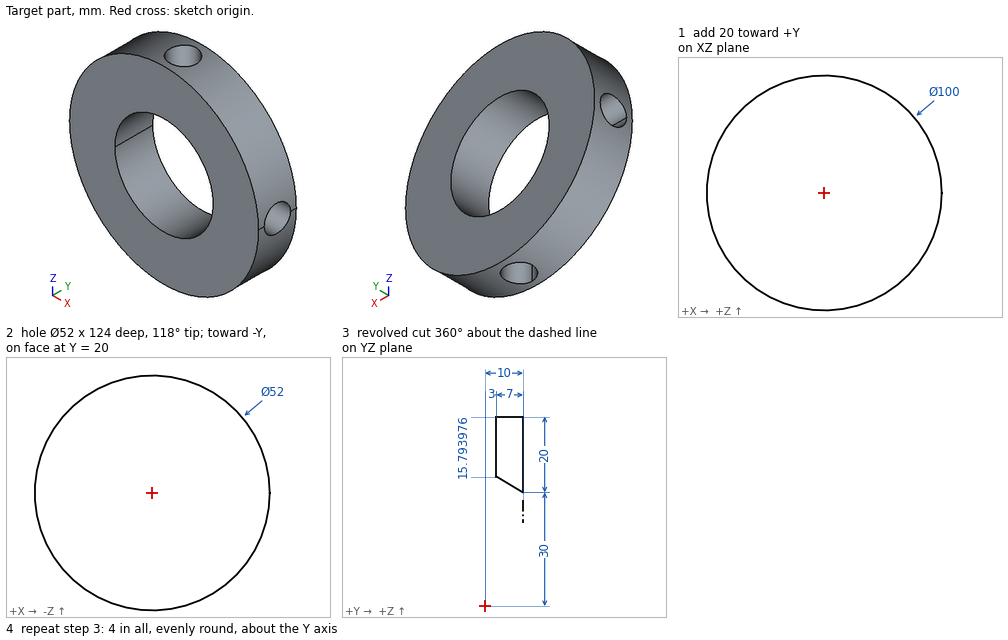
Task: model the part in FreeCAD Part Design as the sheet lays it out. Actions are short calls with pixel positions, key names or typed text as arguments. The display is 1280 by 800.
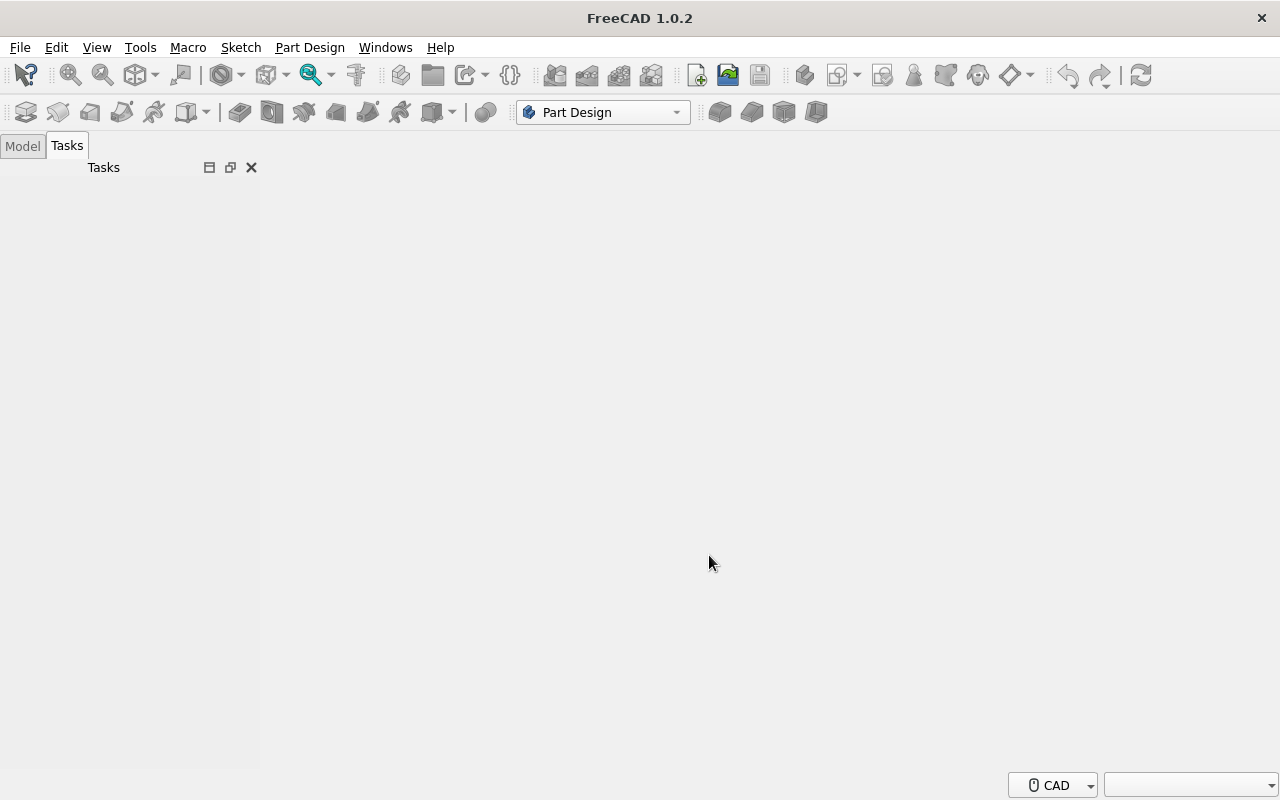
key(ctrl+n)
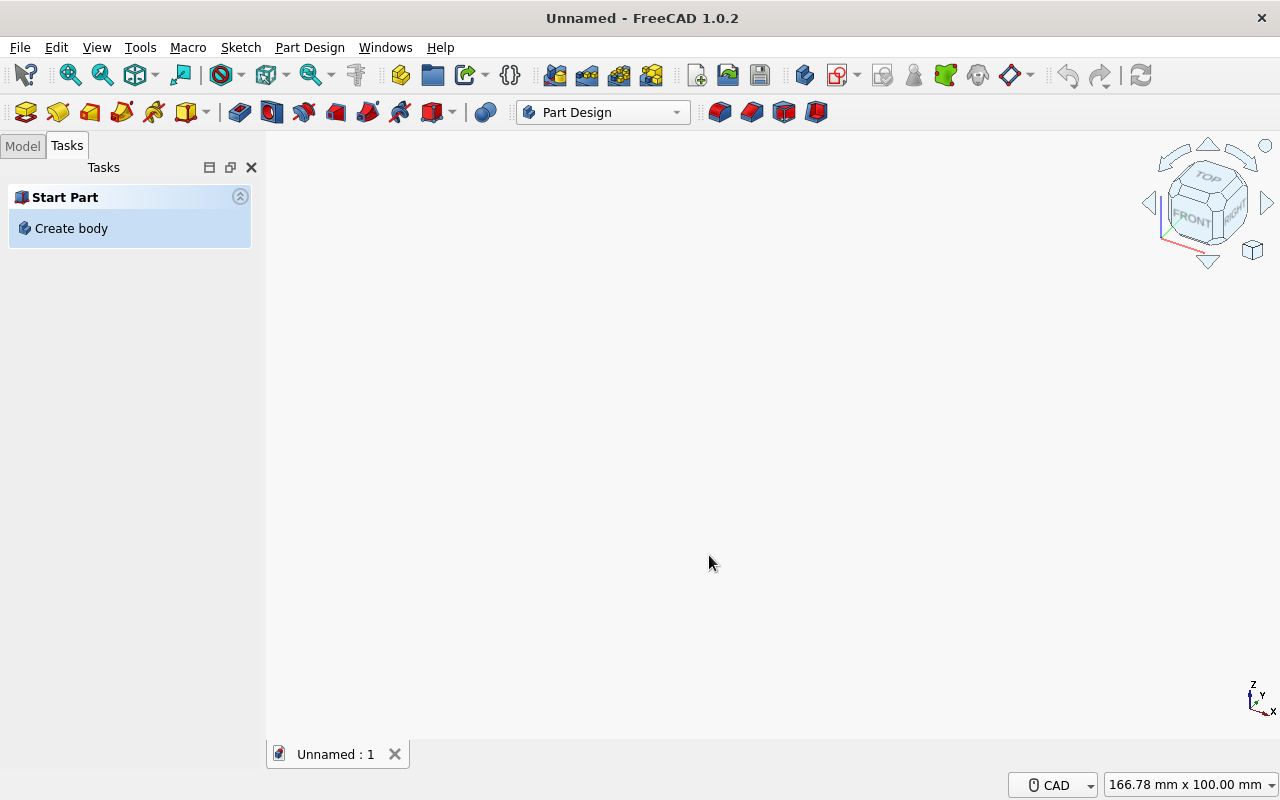
click(838, 76)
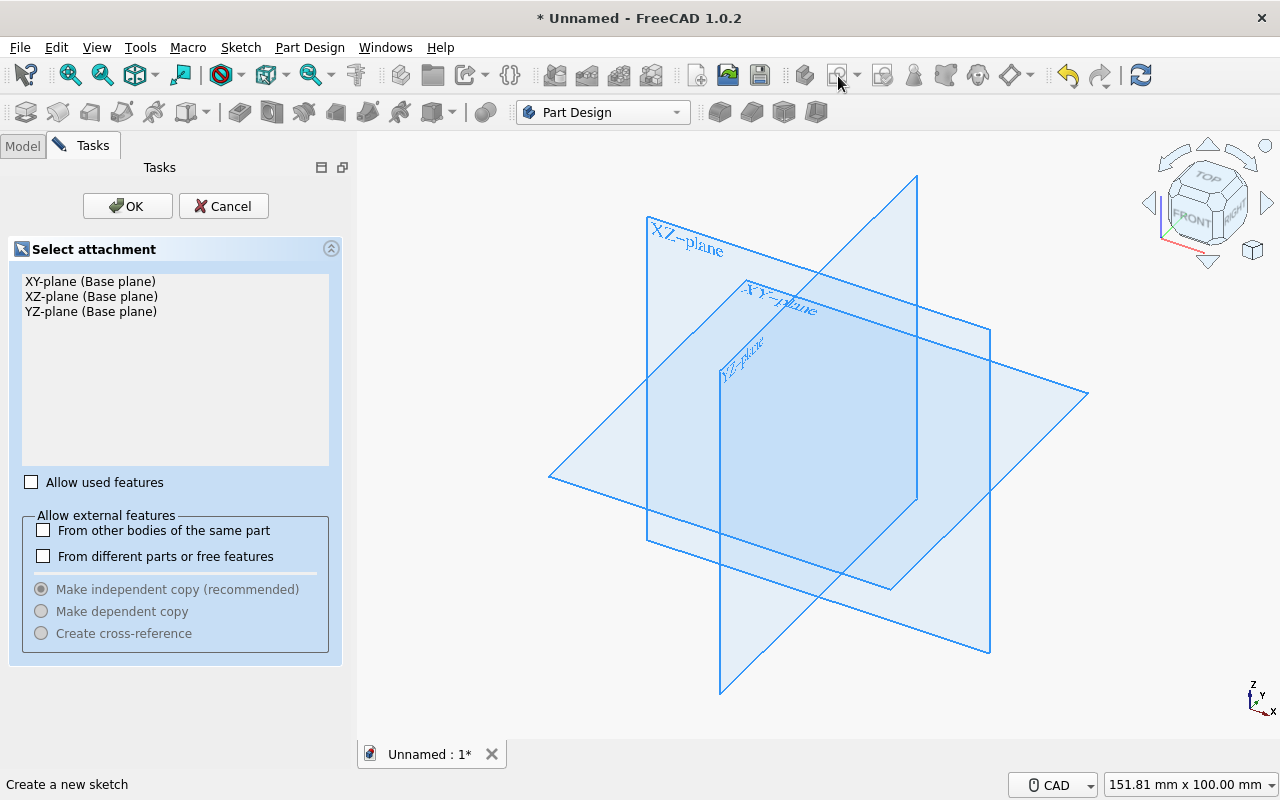
click(82, 296)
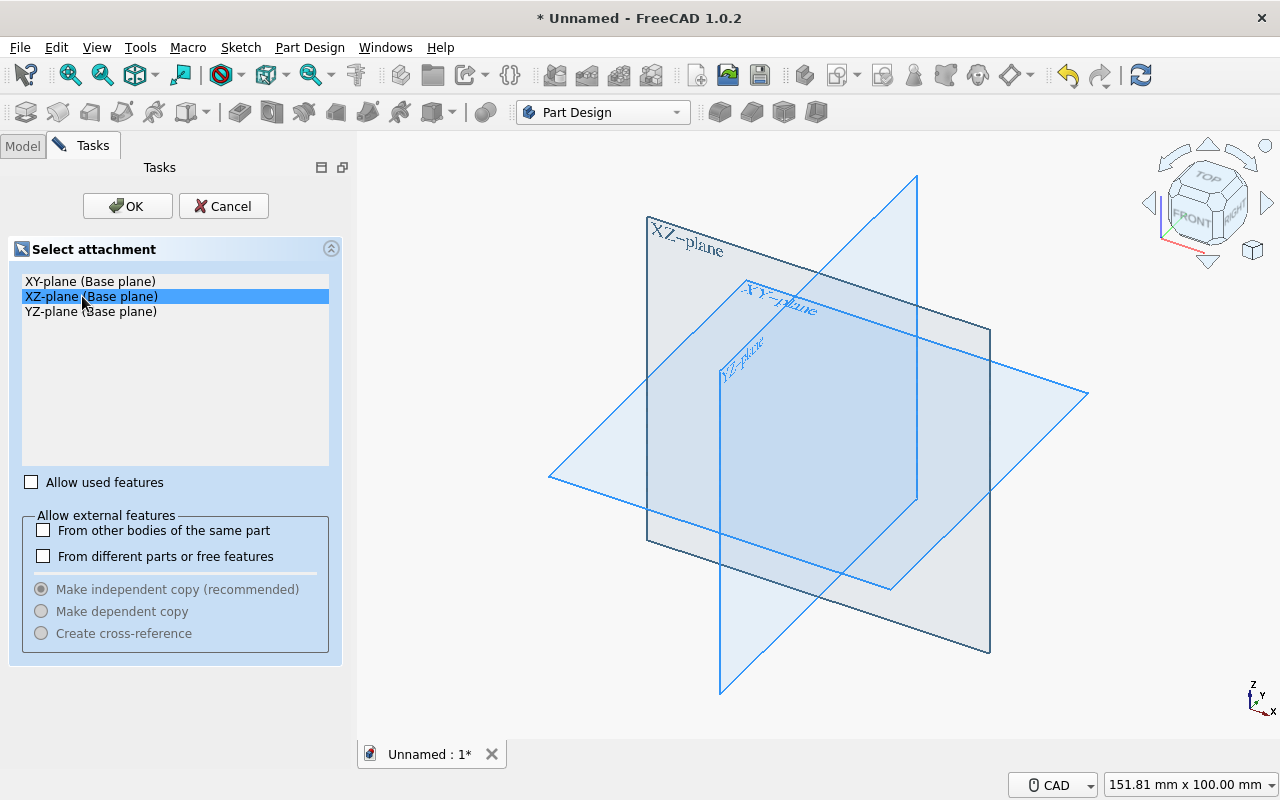
click(128, 206)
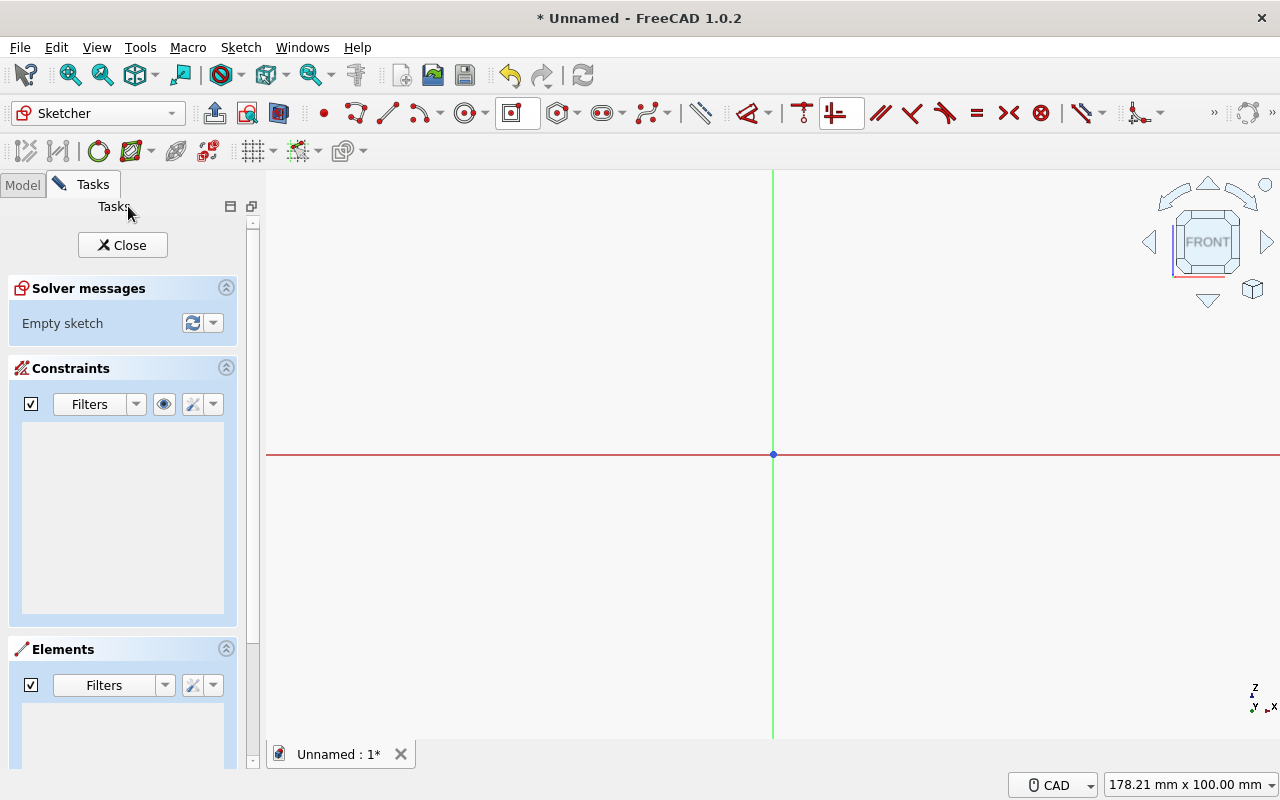
scroll(565, 455, down, 2)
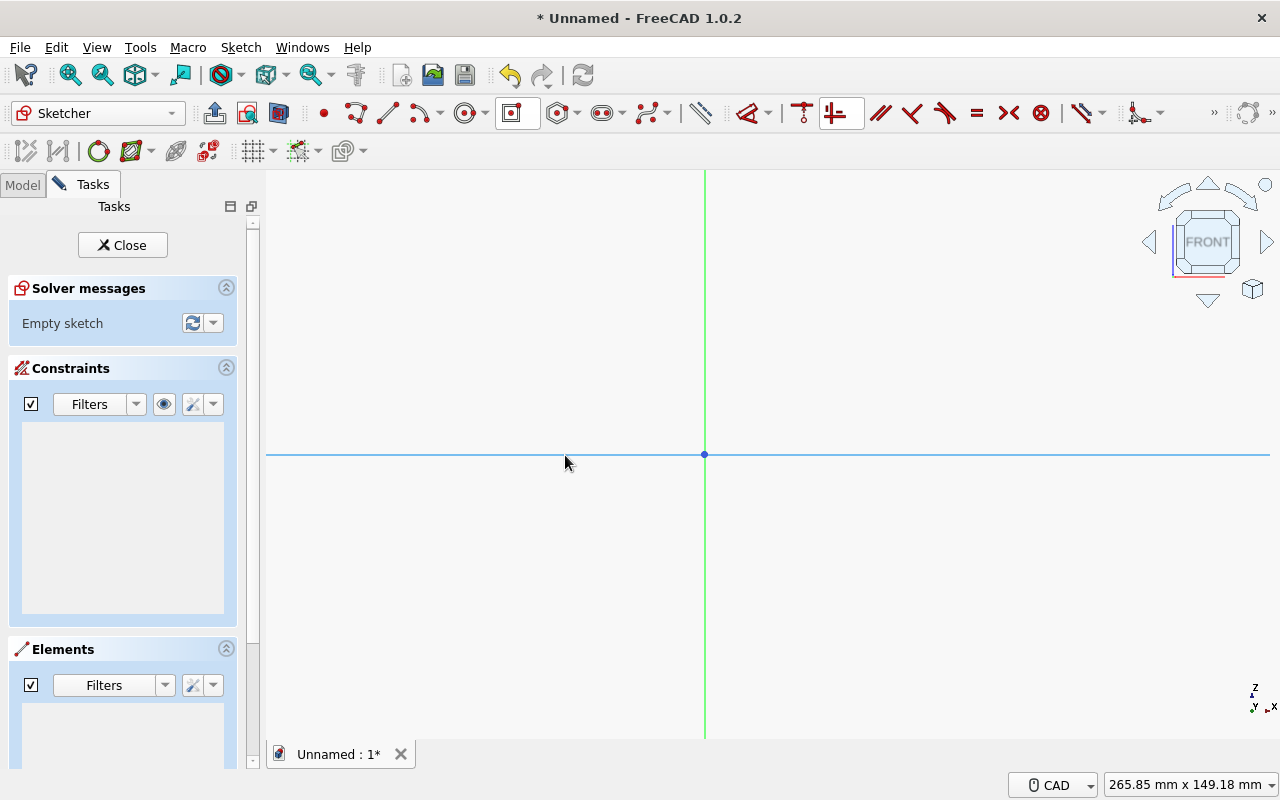
key(g)
key(c)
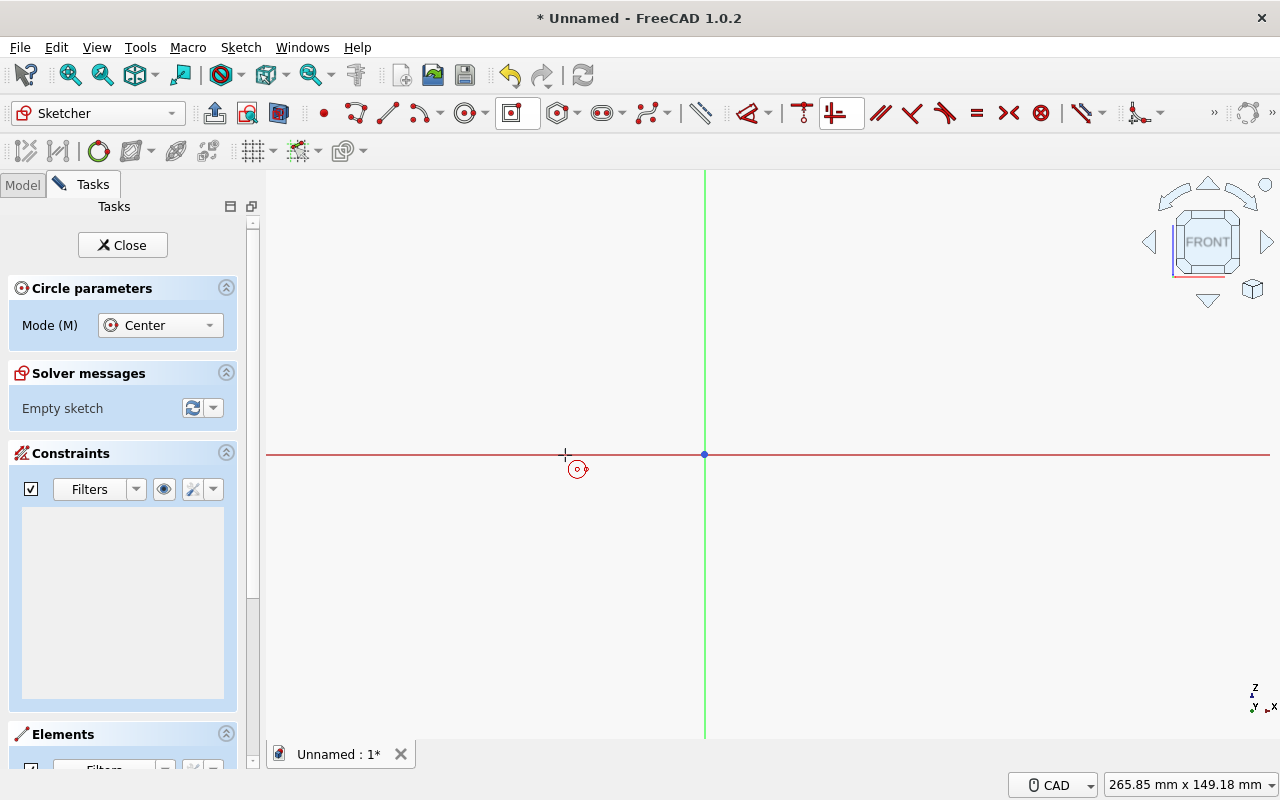
click(705, 455)
move(839, 320)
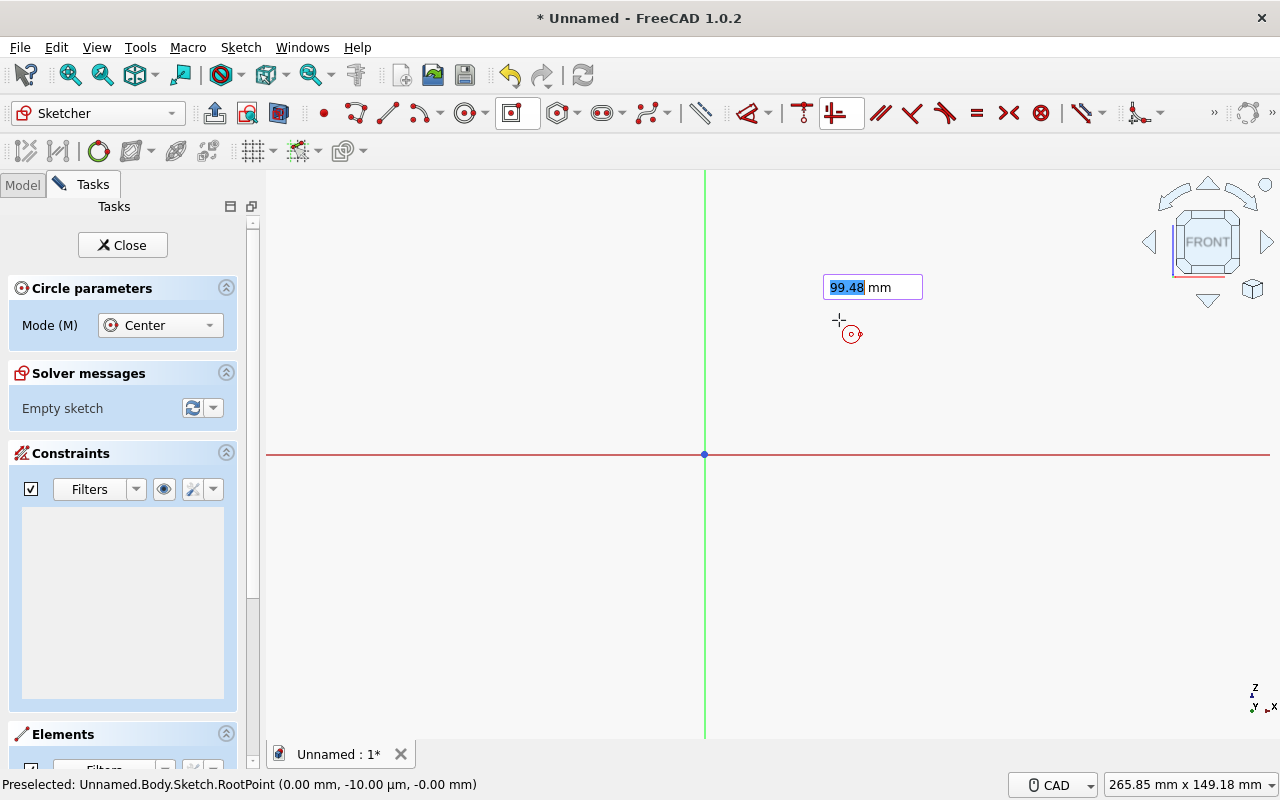
text(100)
key(Return)
key(Escape)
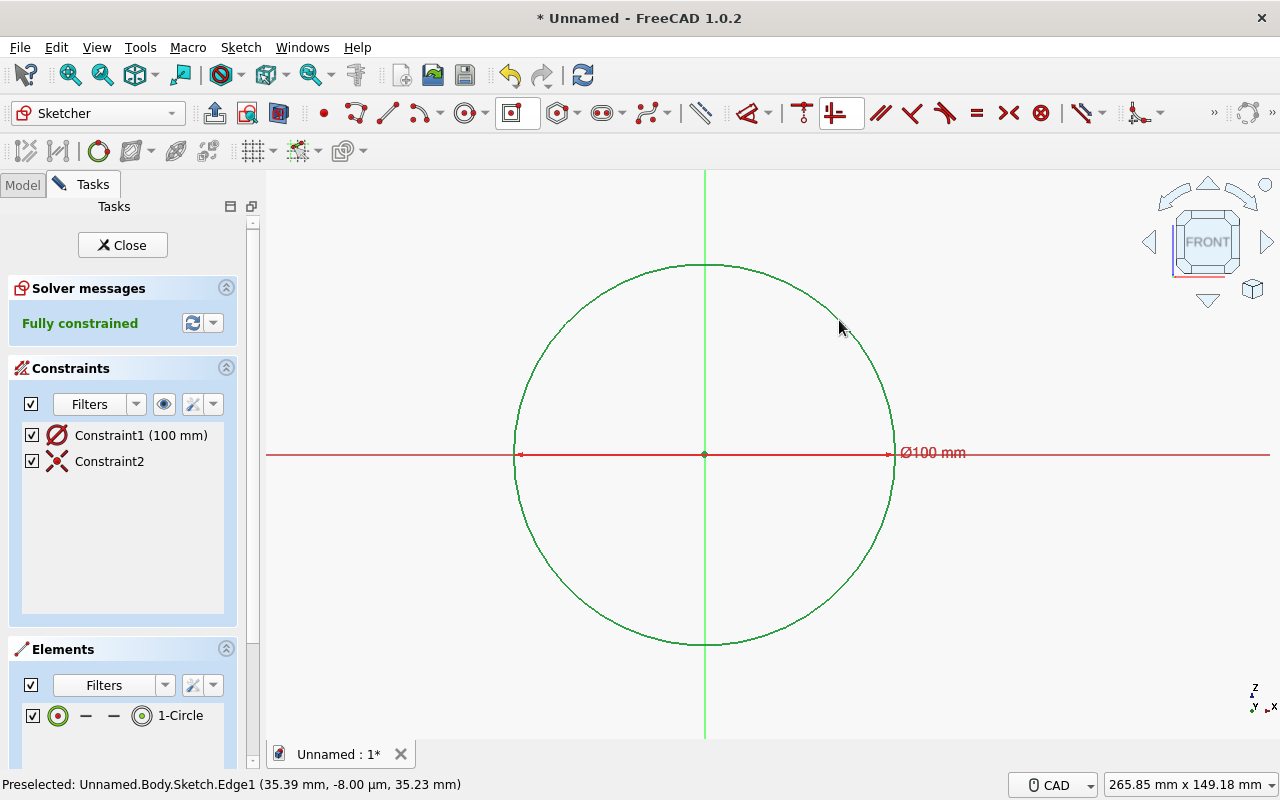
click(123, 245)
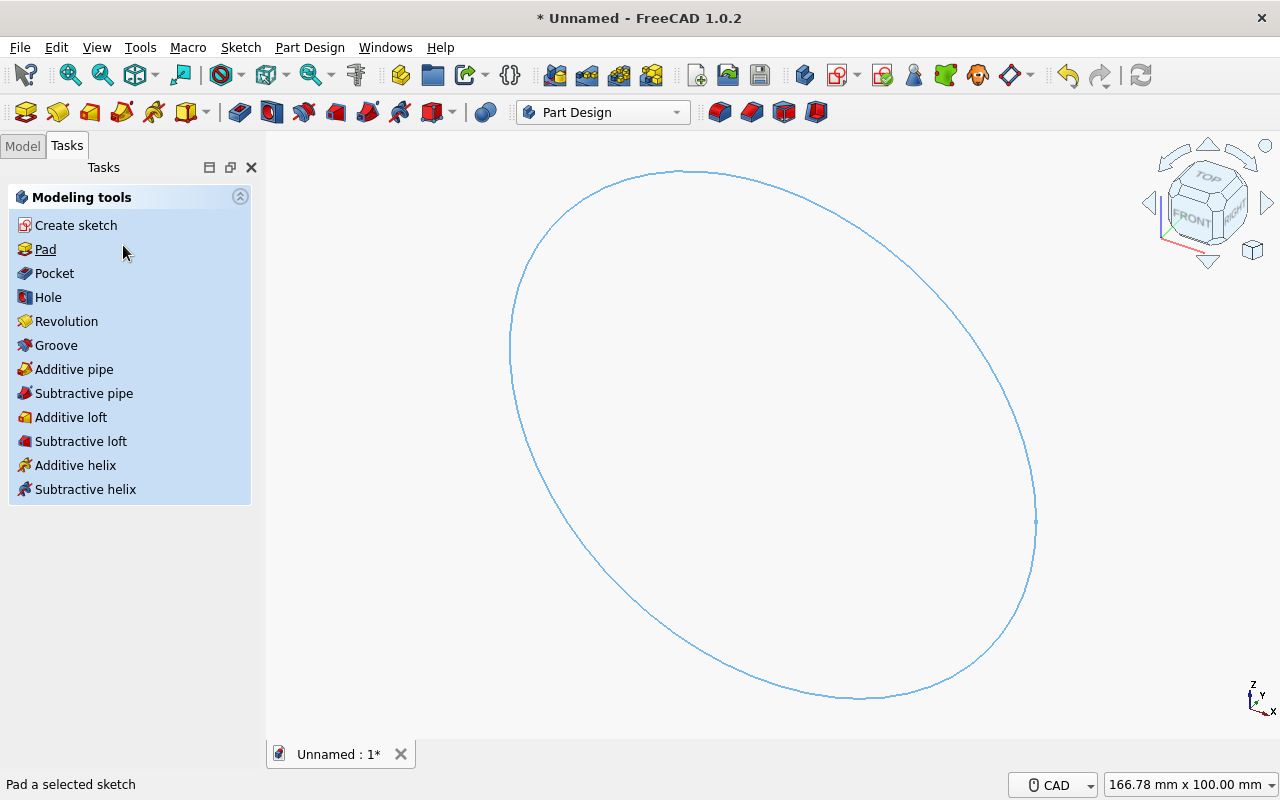
click(26, 112)